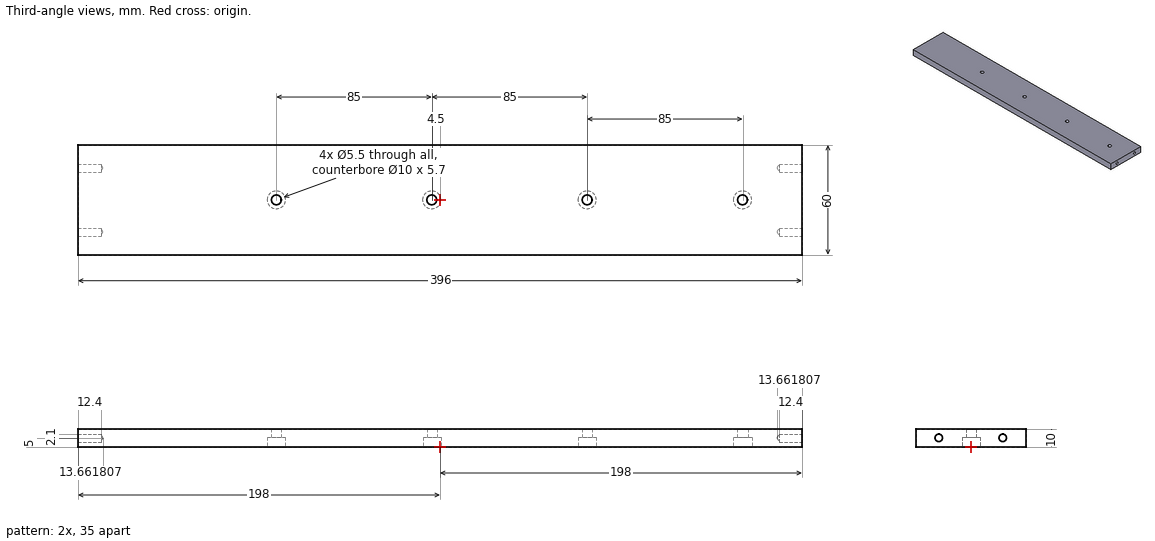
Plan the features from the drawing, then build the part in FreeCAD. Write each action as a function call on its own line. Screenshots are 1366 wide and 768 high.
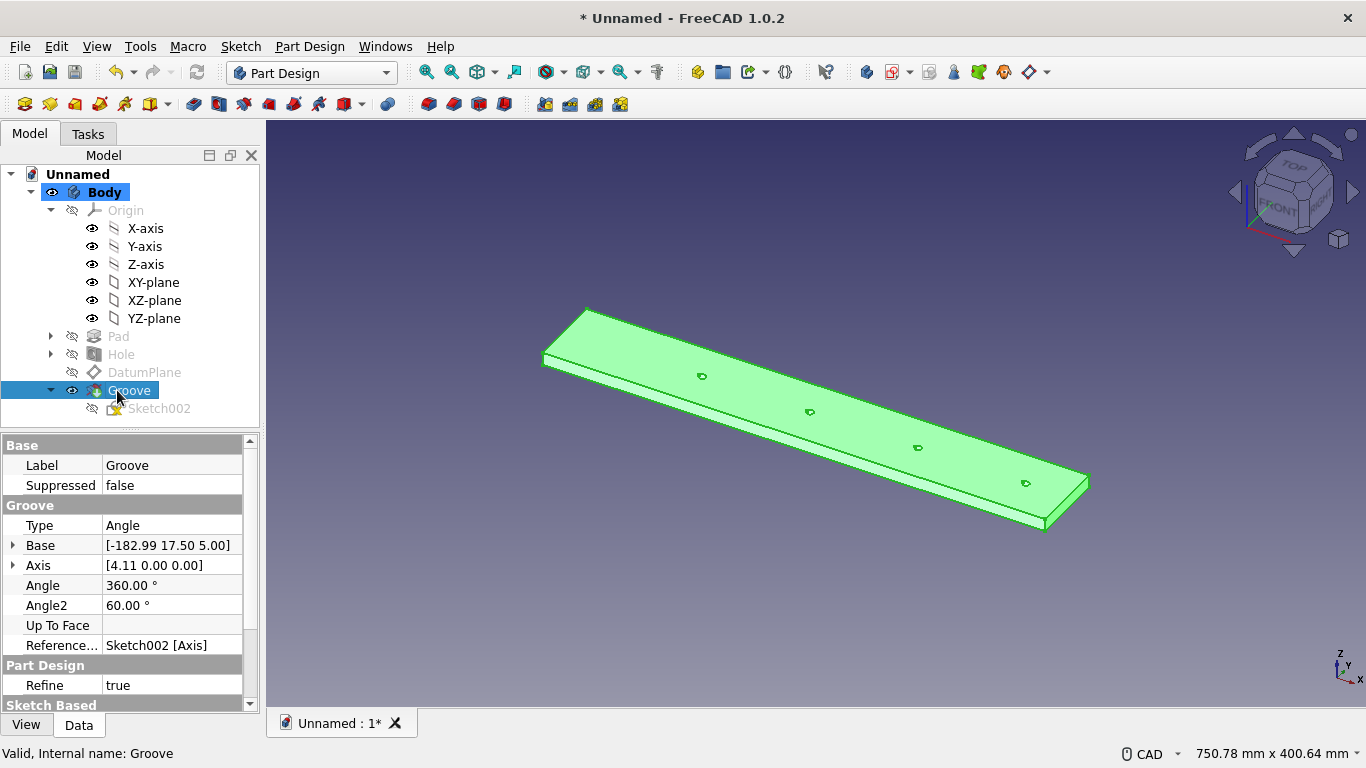
click(570, 104)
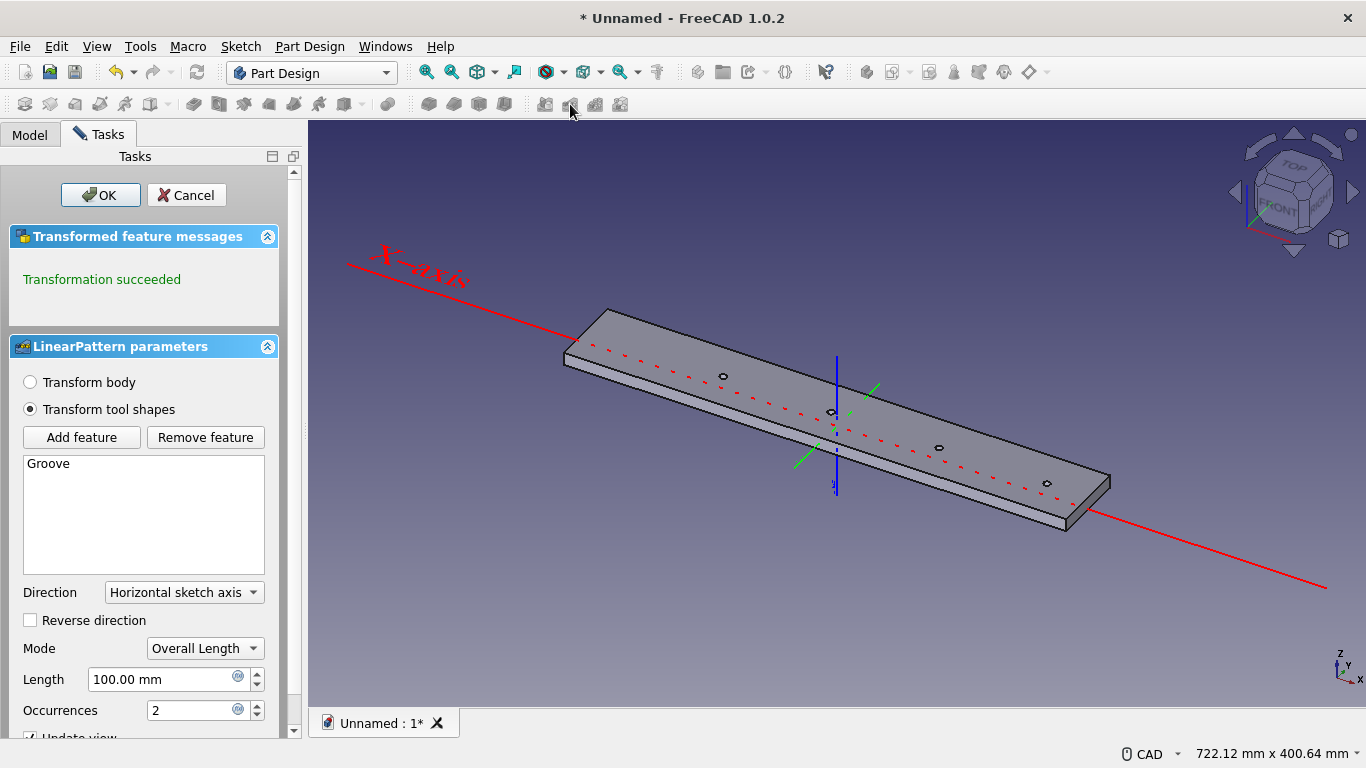
click(185, 592)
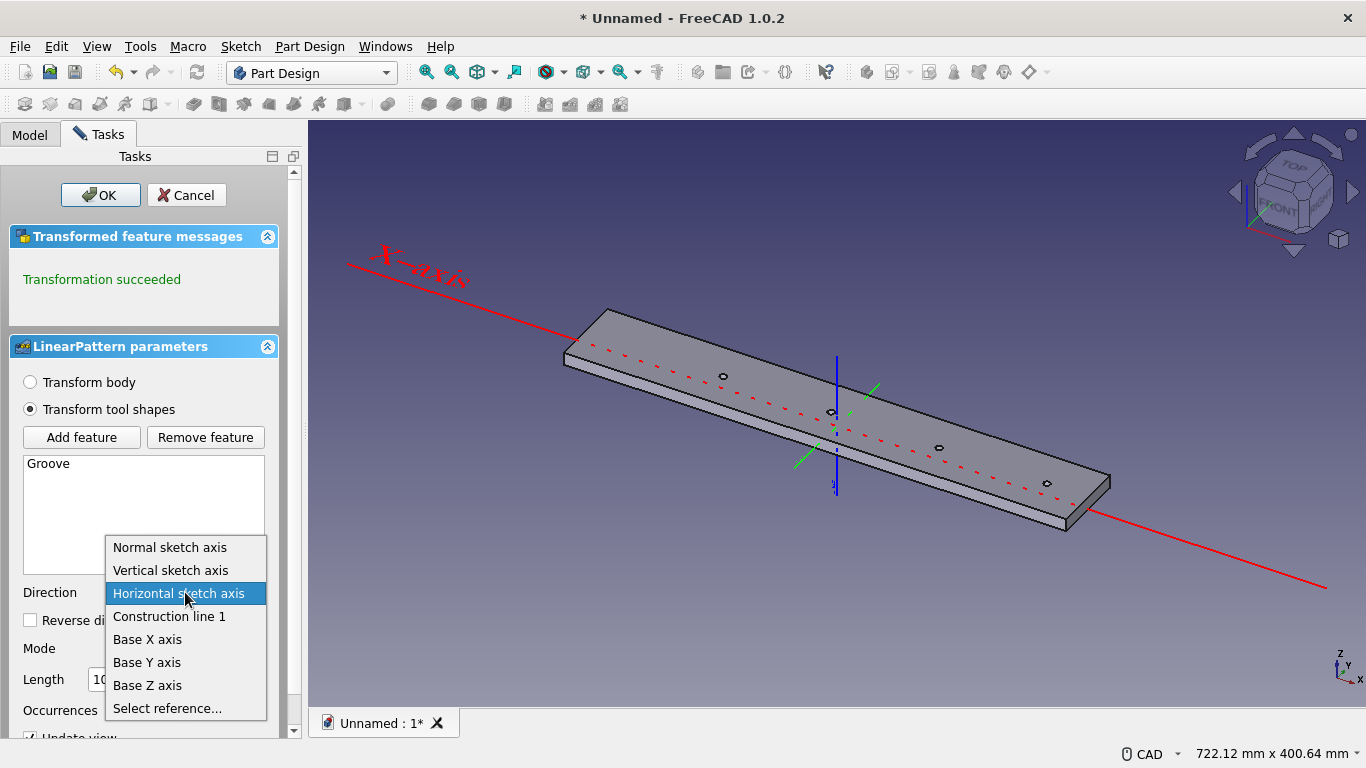
click(184, 662)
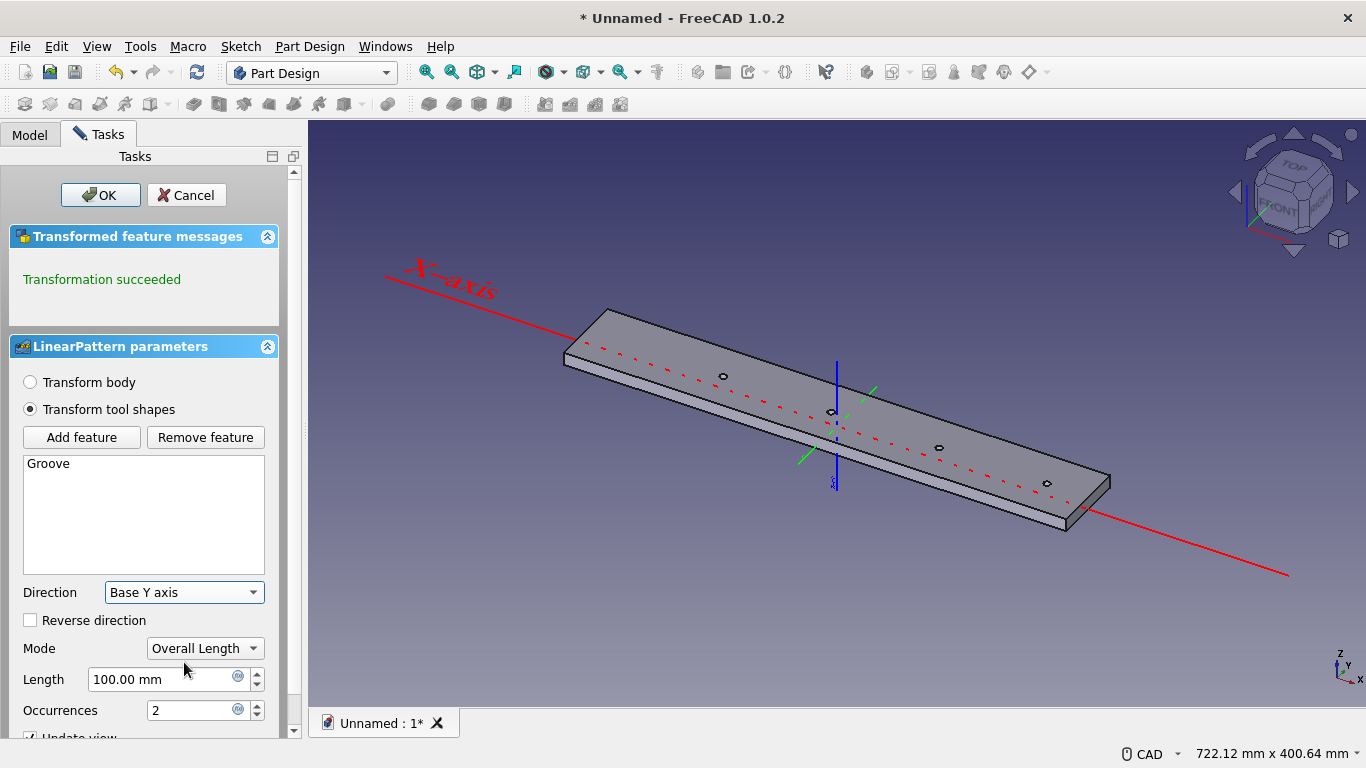
click(206, 648)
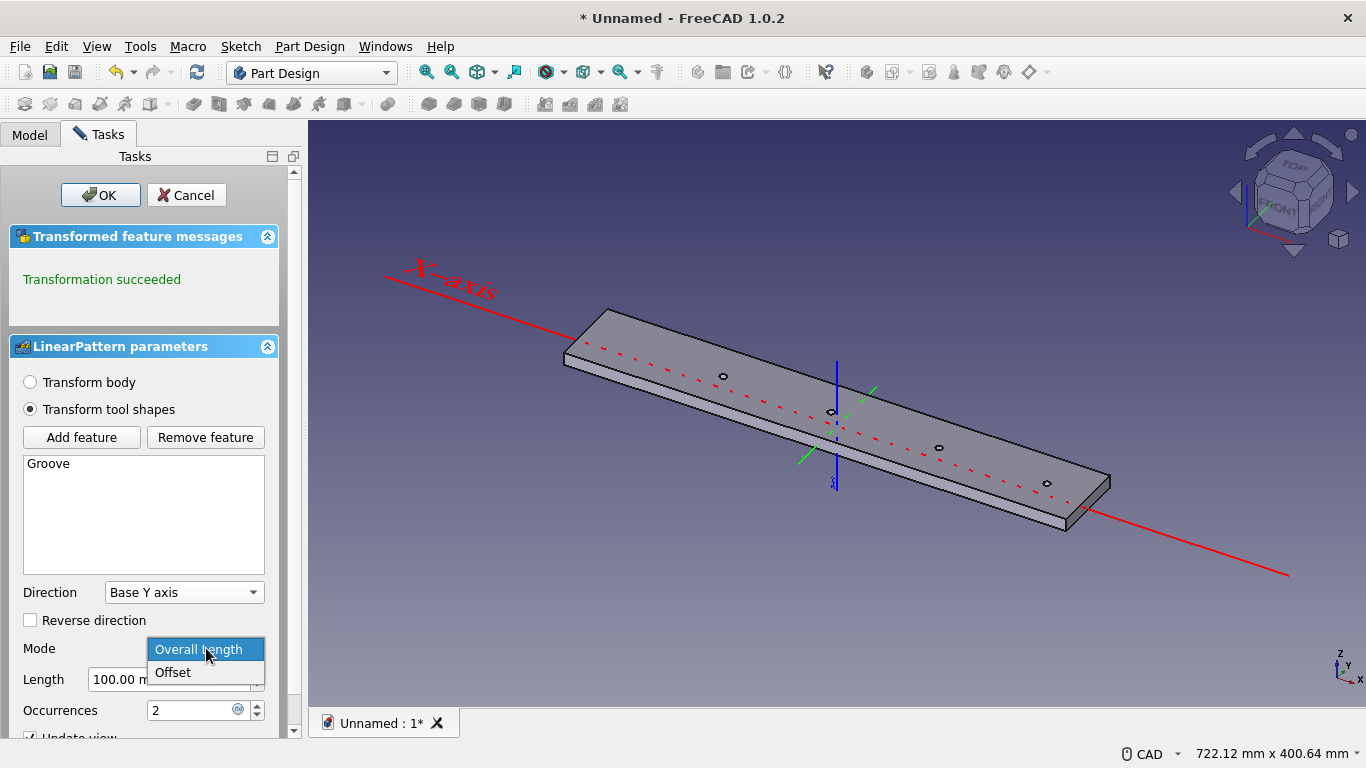
click(204, 672)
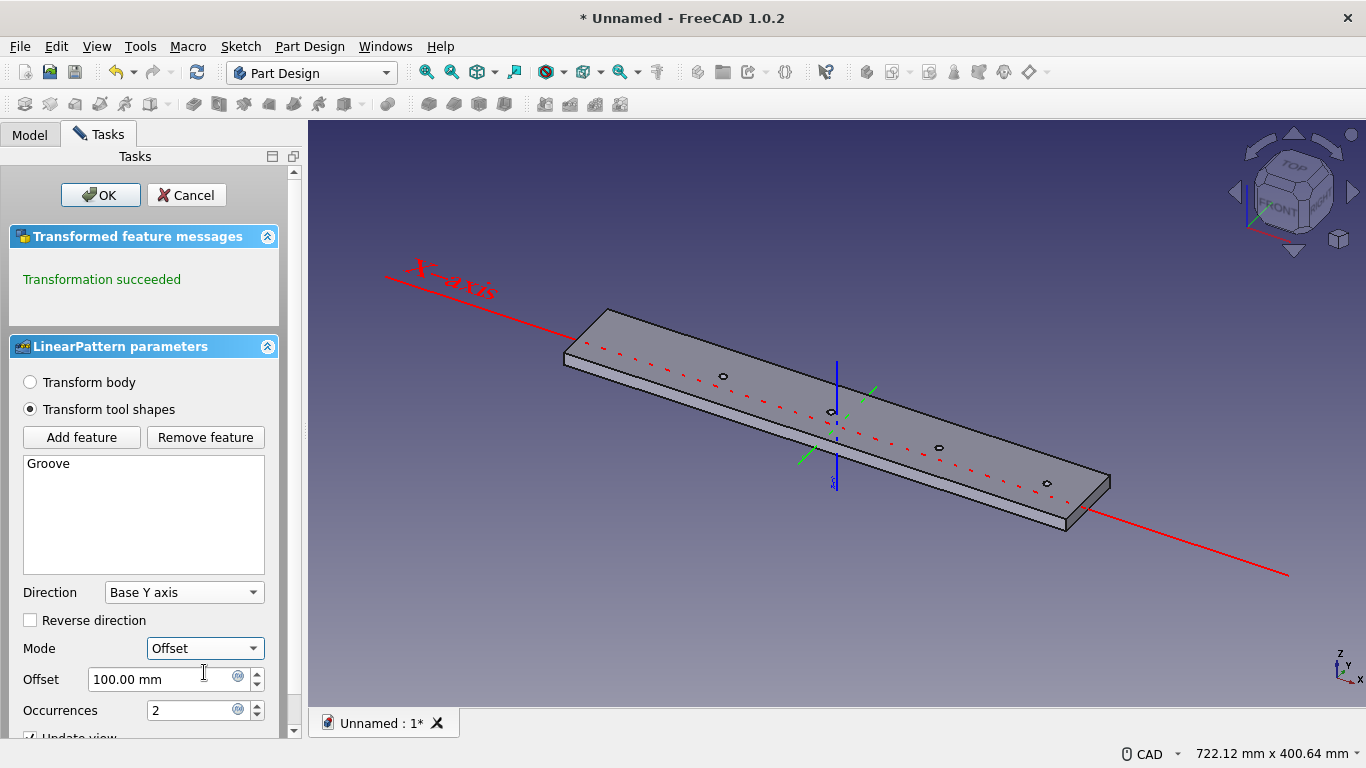
triple_click(170, 680)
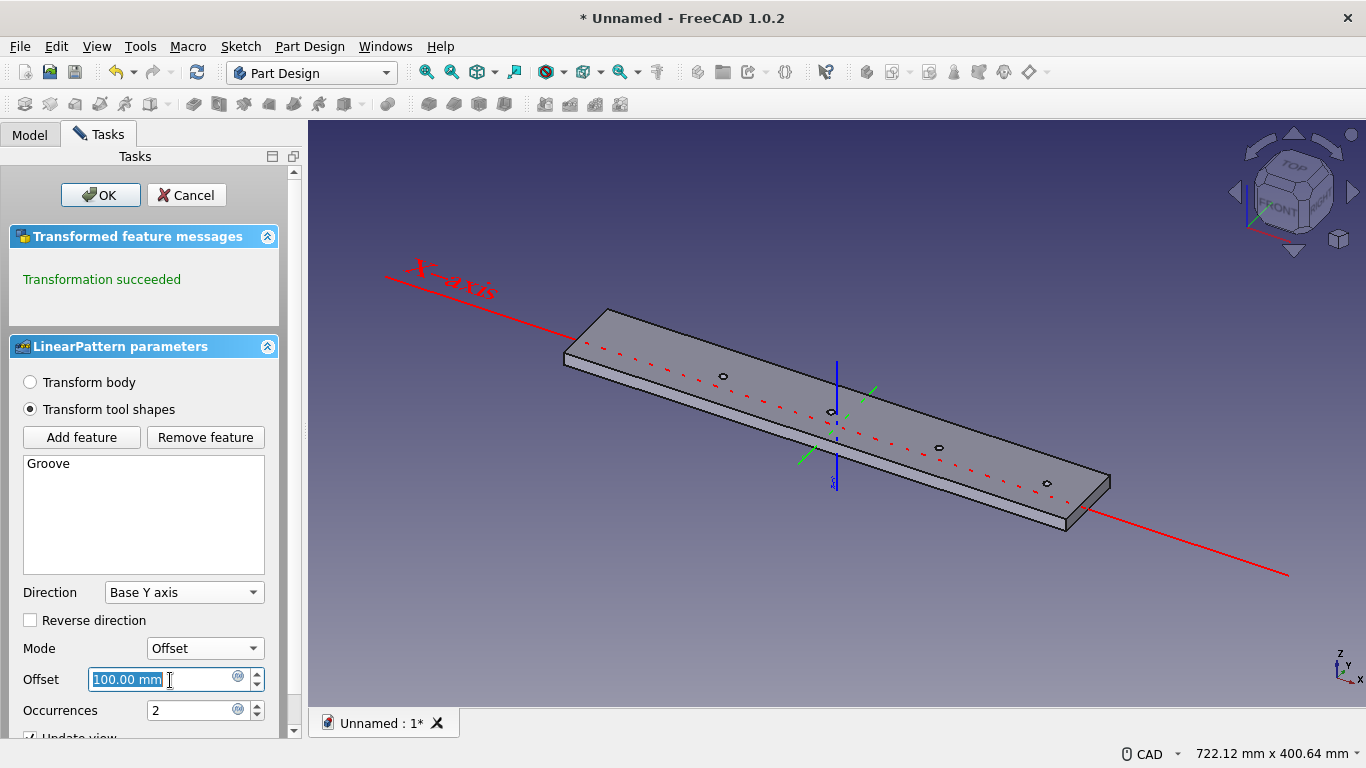
text(35)
key(Tab)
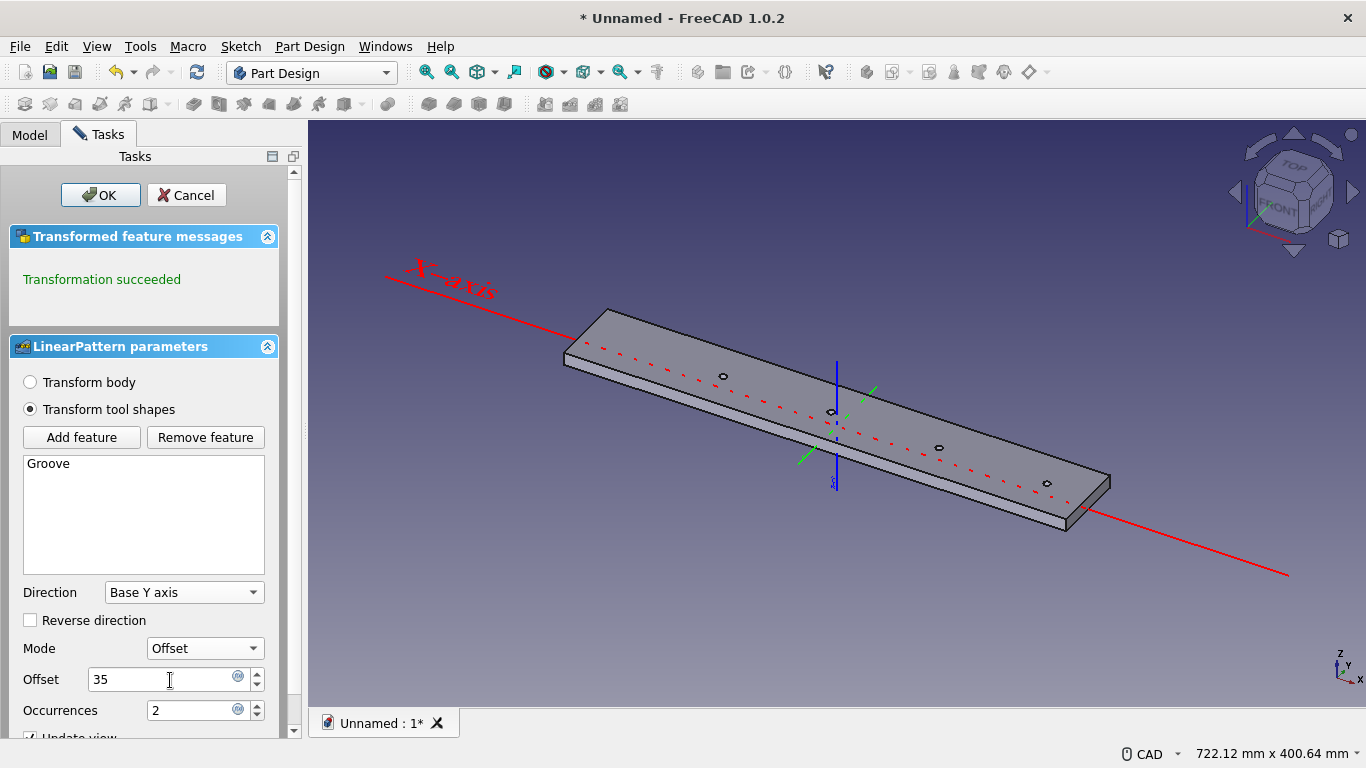
triple_click(199, 710)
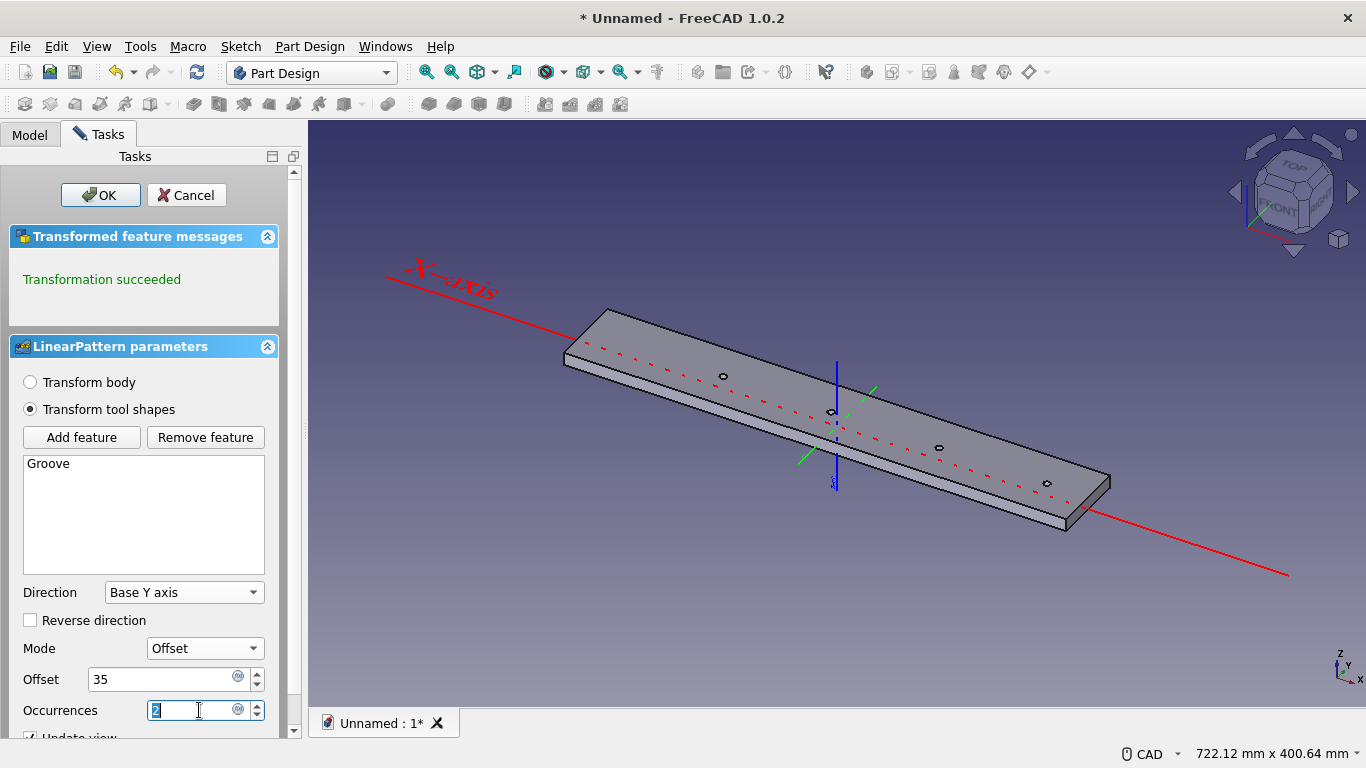
text(2)
key(Tab)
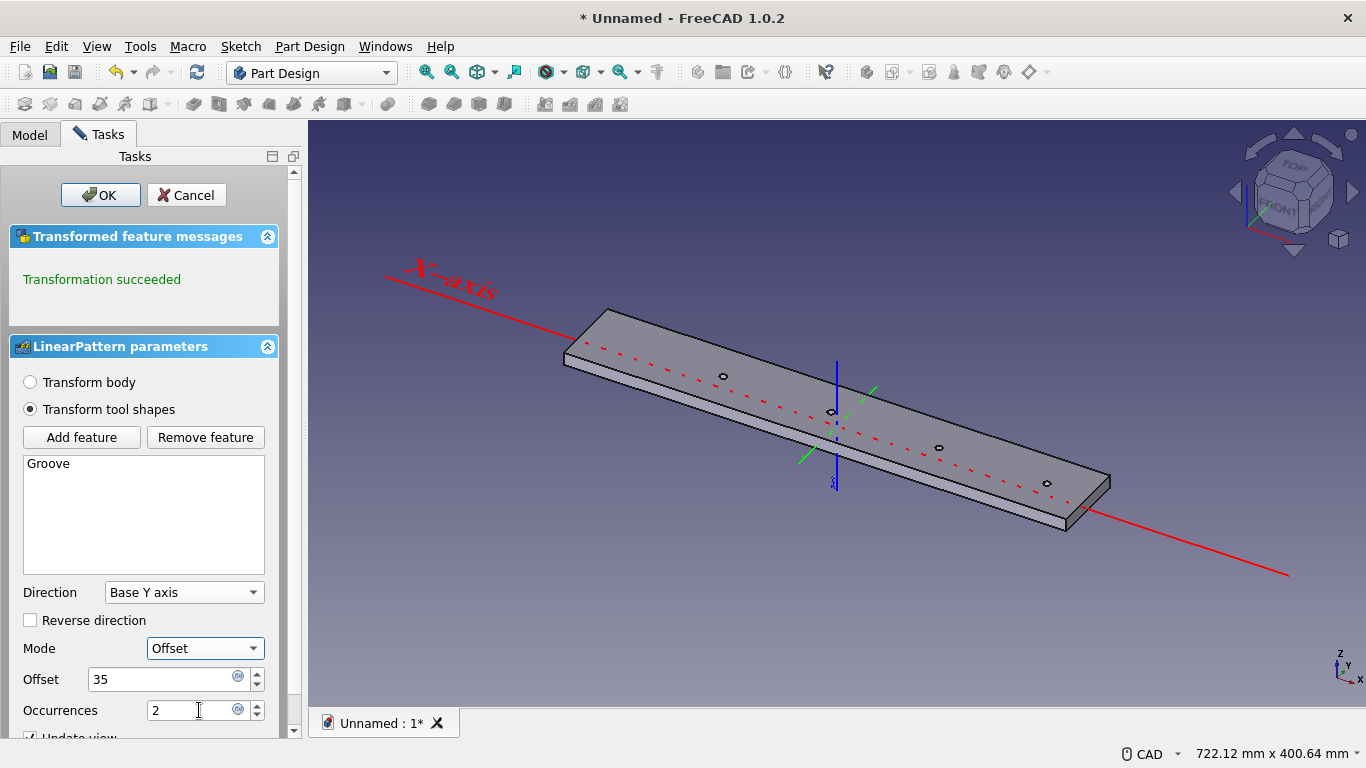
click(31, 620)